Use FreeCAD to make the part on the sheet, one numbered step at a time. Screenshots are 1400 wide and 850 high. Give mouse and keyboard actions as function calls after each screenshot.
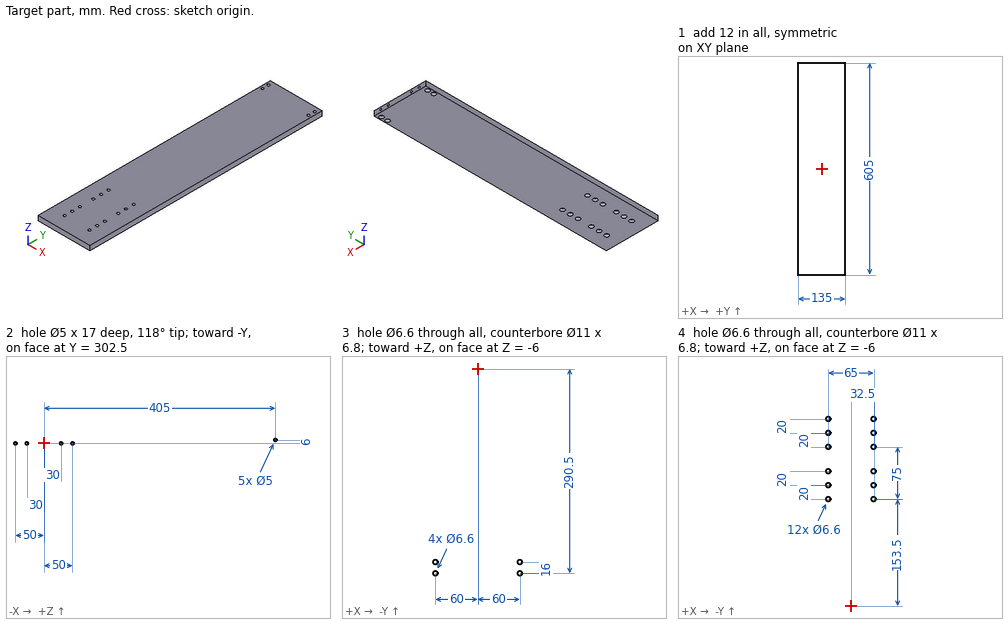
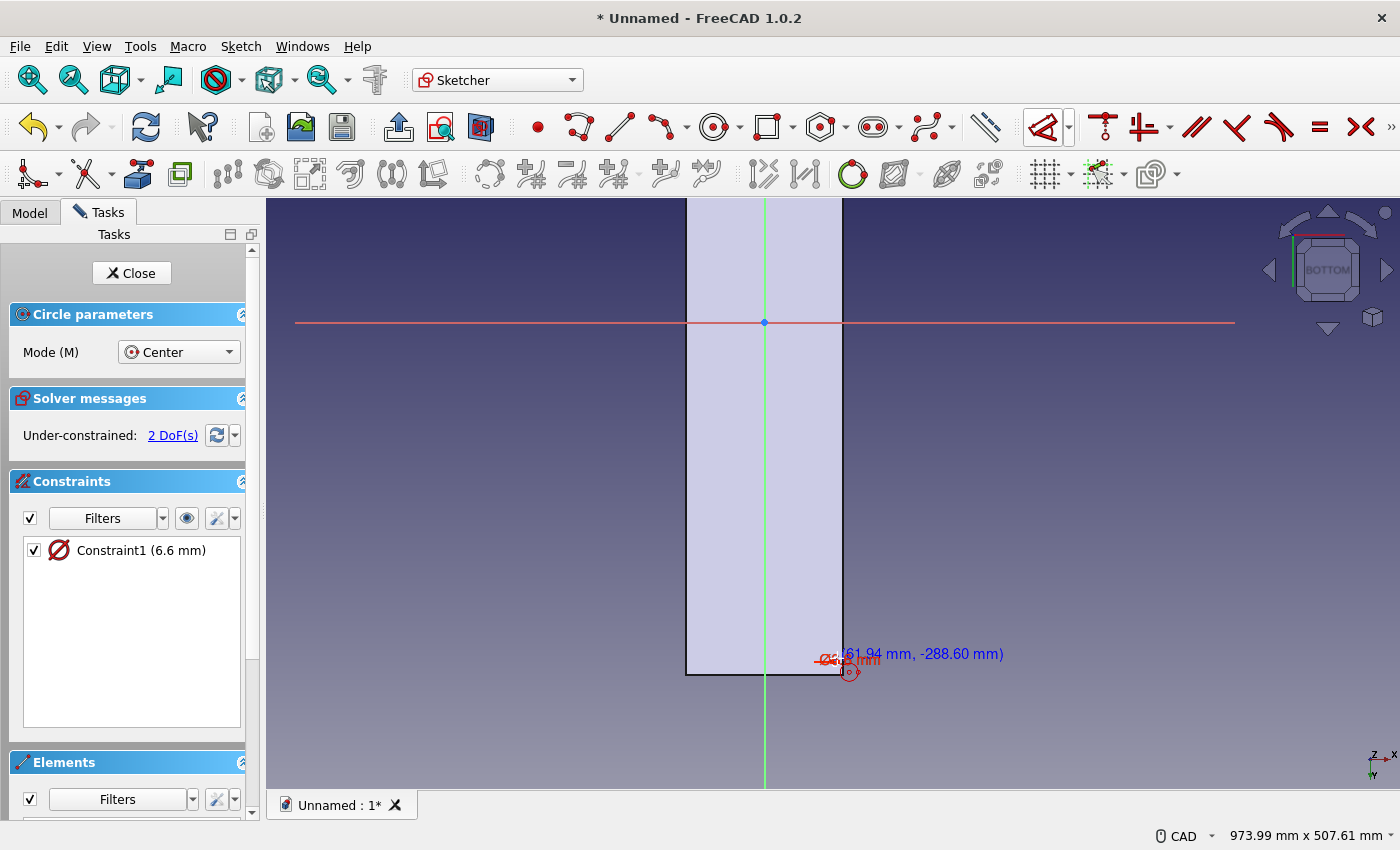
scroll(695, 661, up, 9)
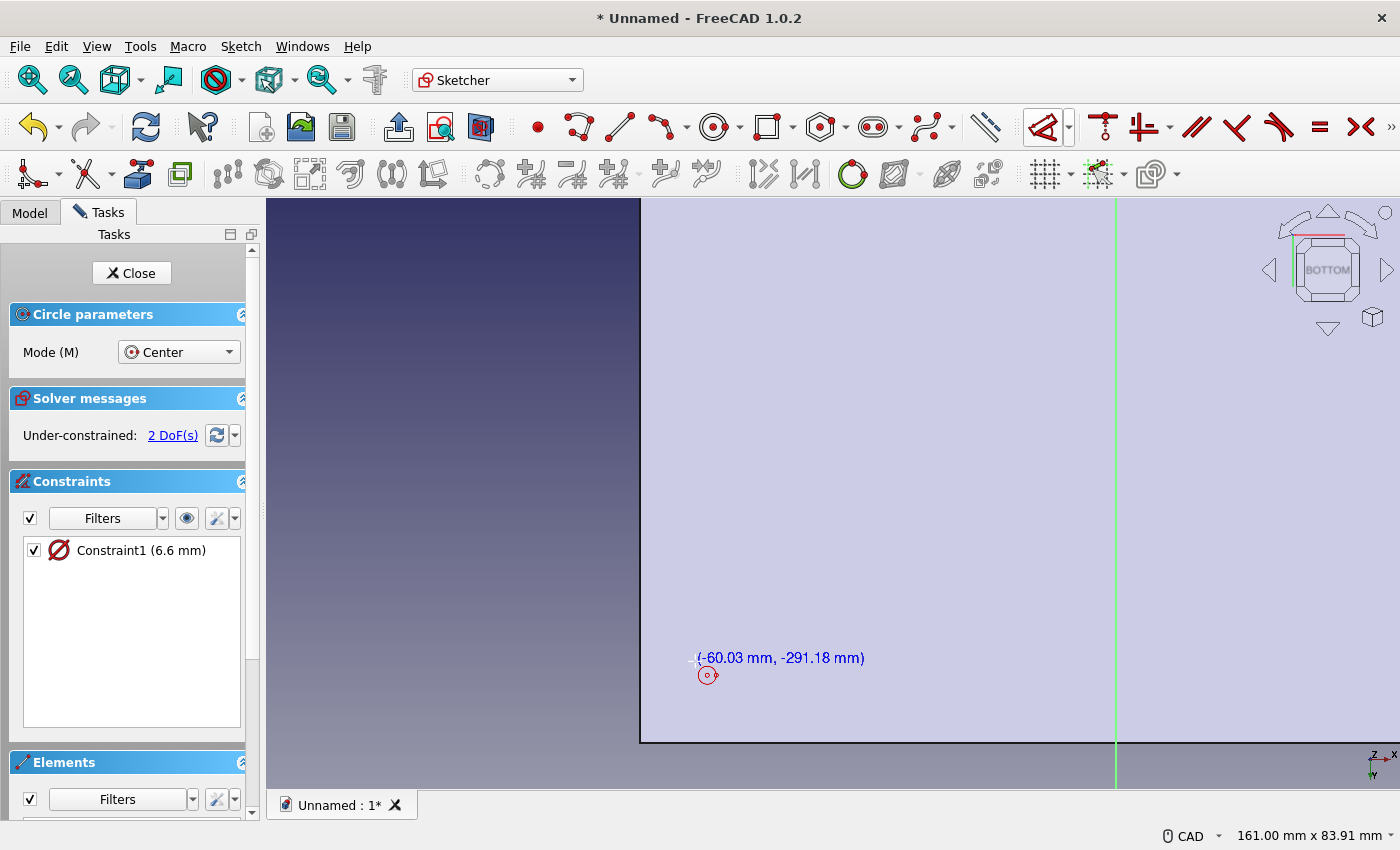
scroll(695, 661, down, 9)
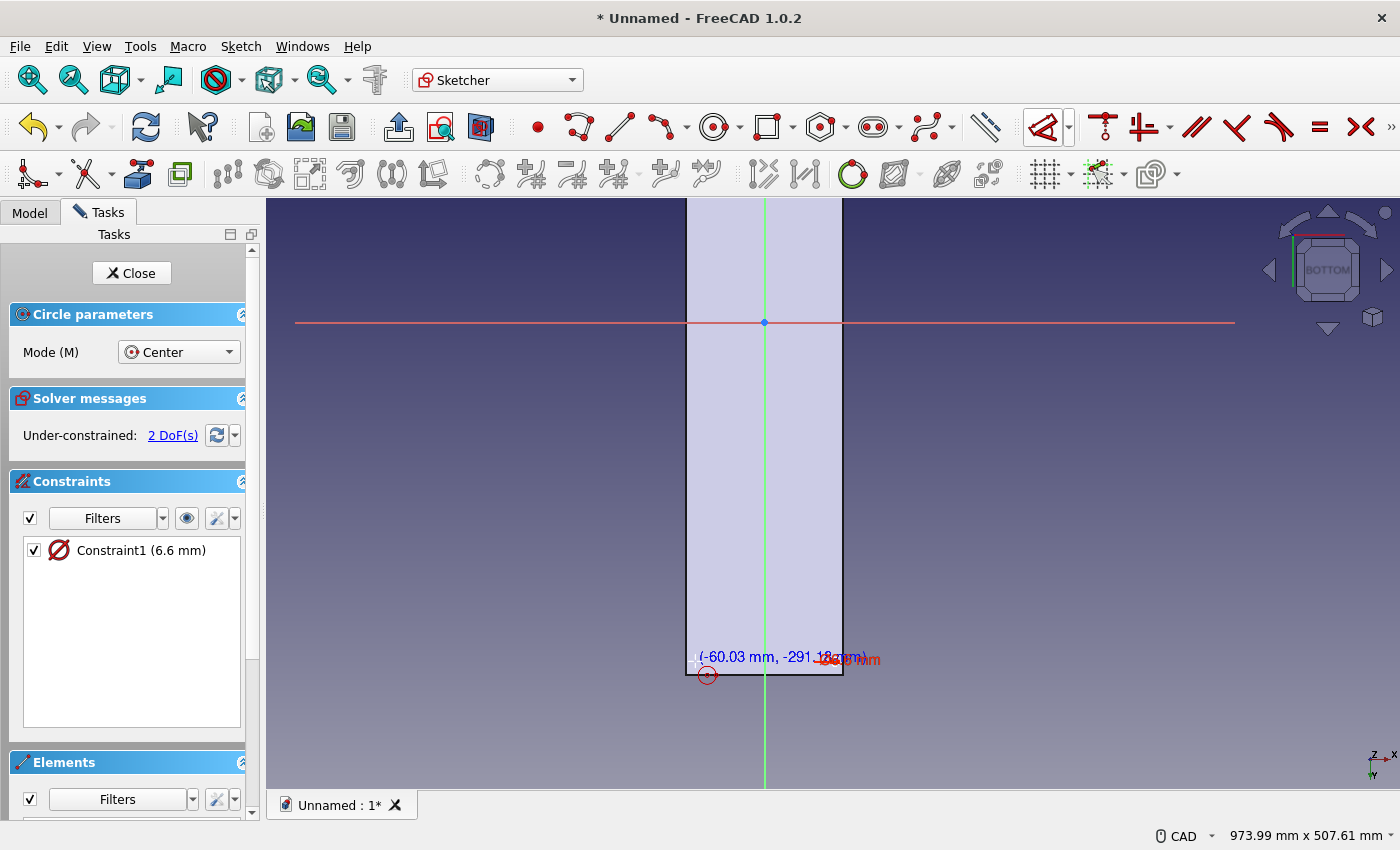
click(695, 661)
move(698, 658)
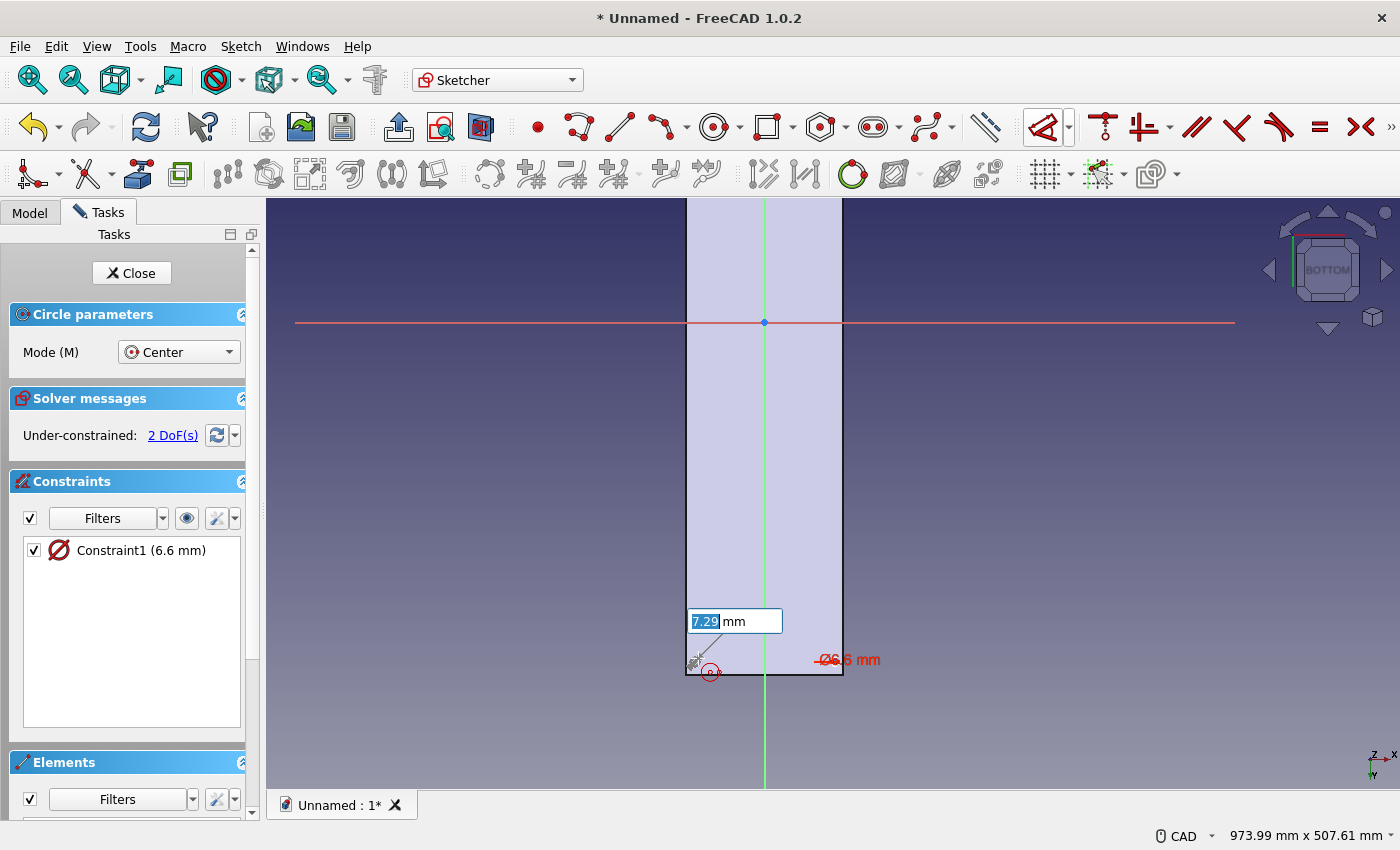
text(6.6)
key(Return)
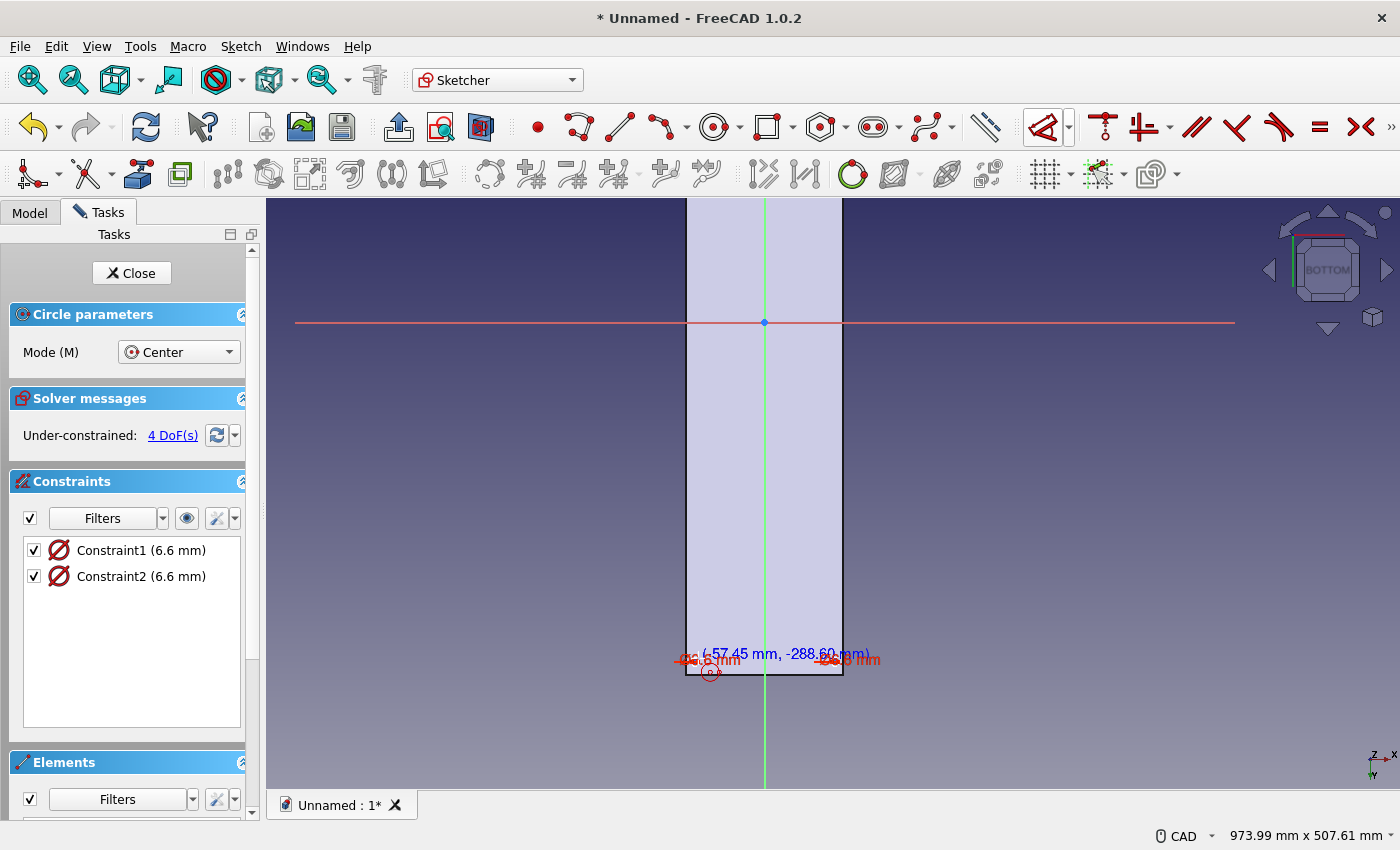
scroll(835, 643, up, 9)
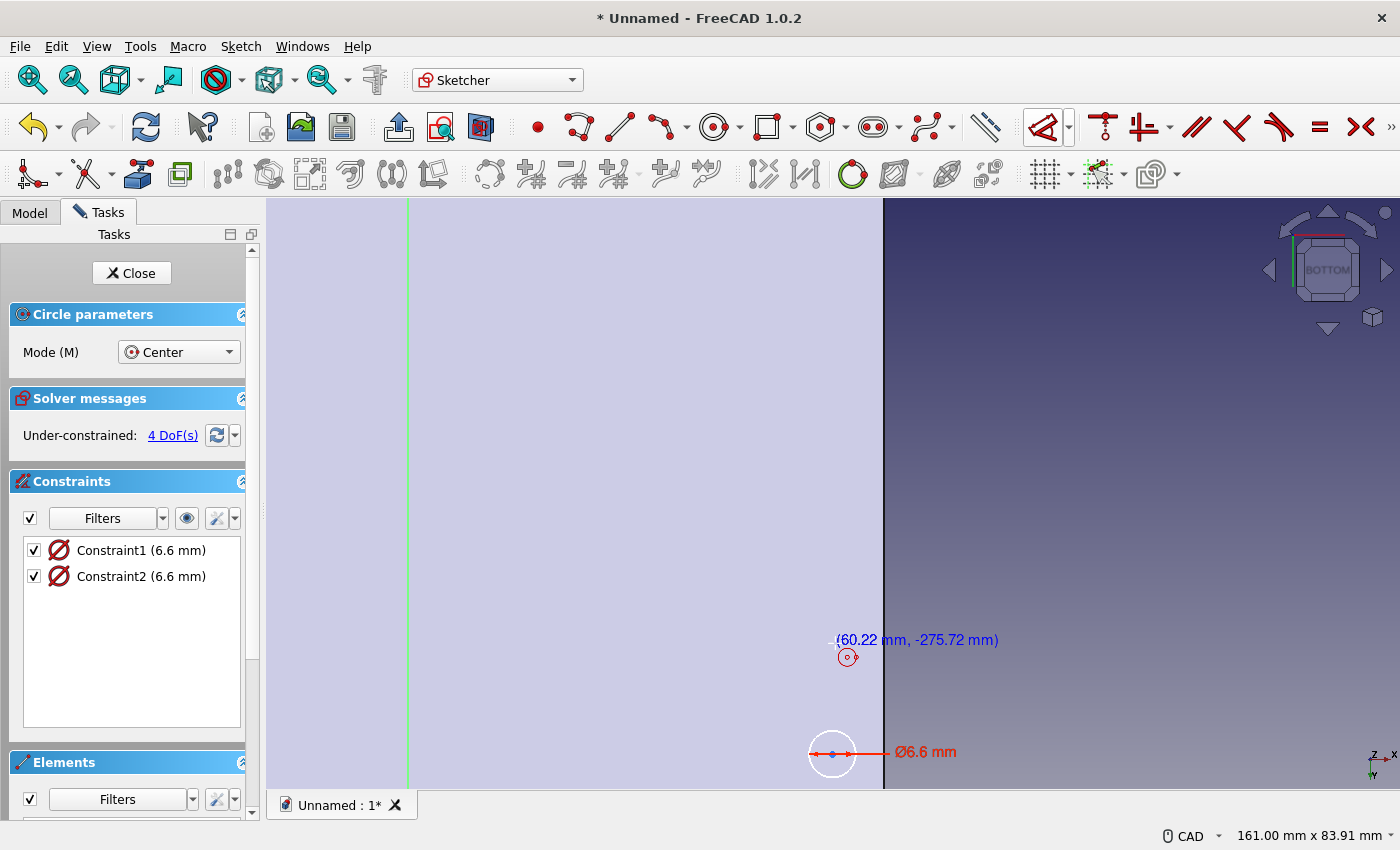
scroll(835, 643, down, 9)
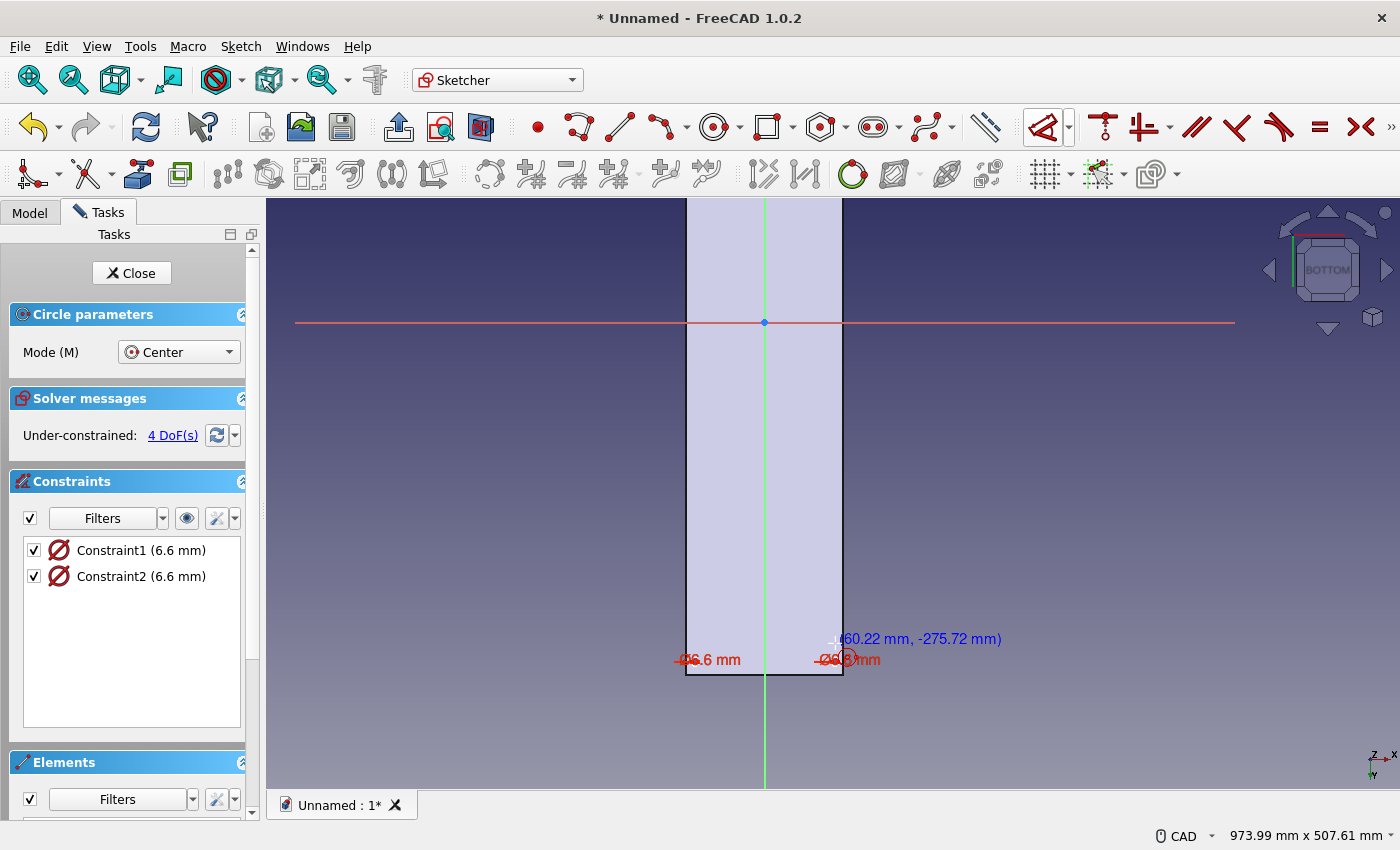
click(835, 643)
move(837, 640)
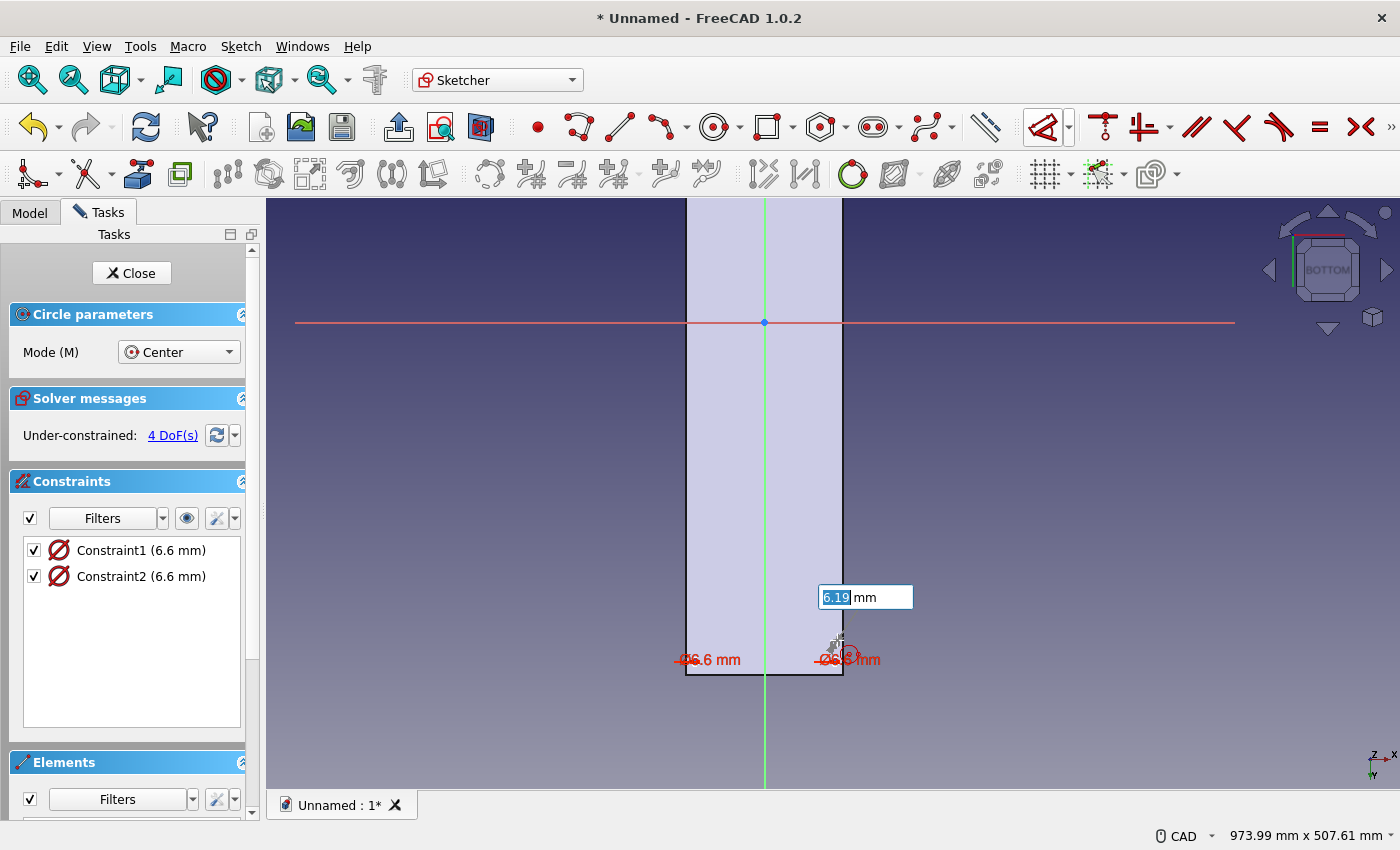
text(6.6)
key(Return)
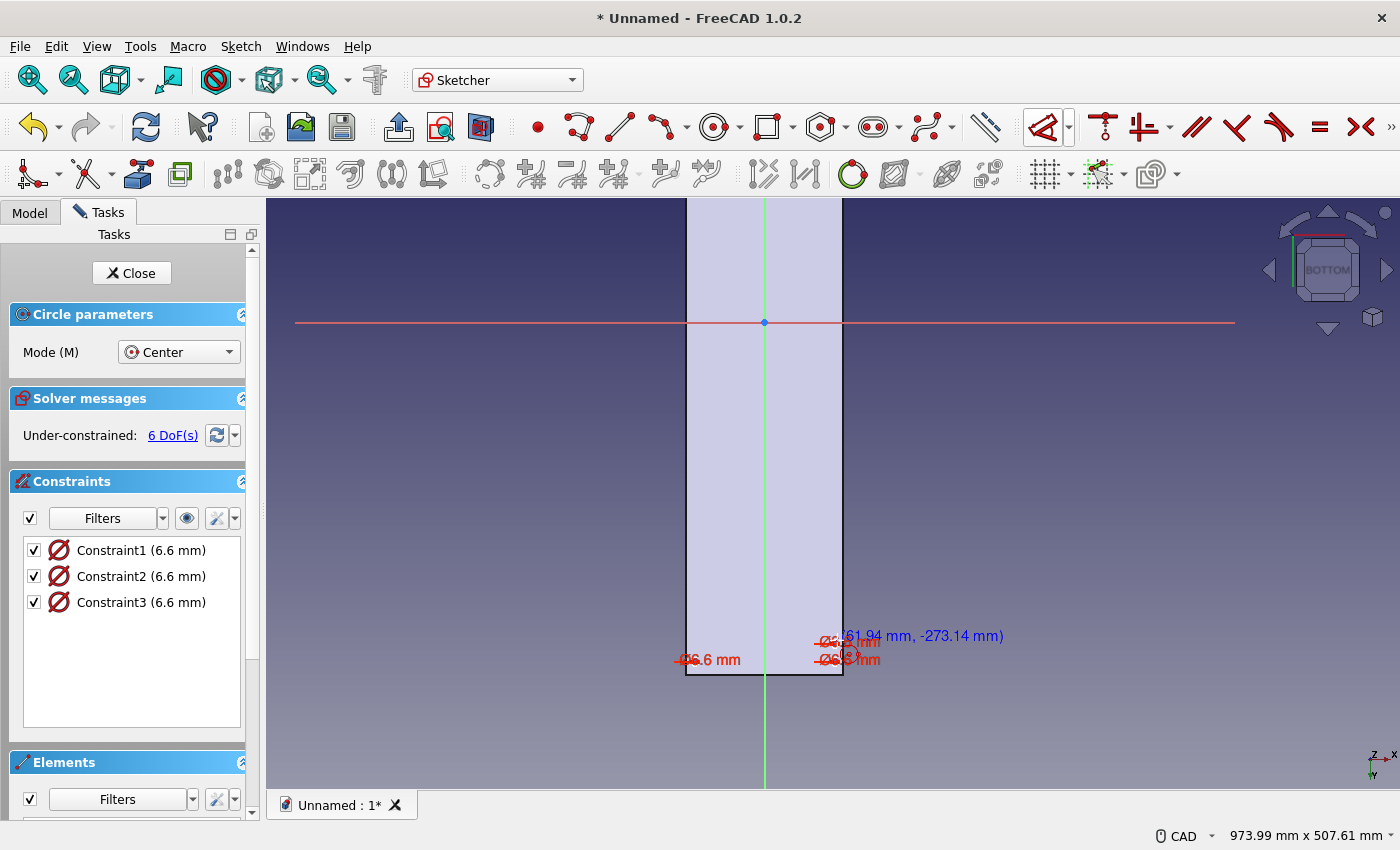
scroll(695, 643, up, 9)